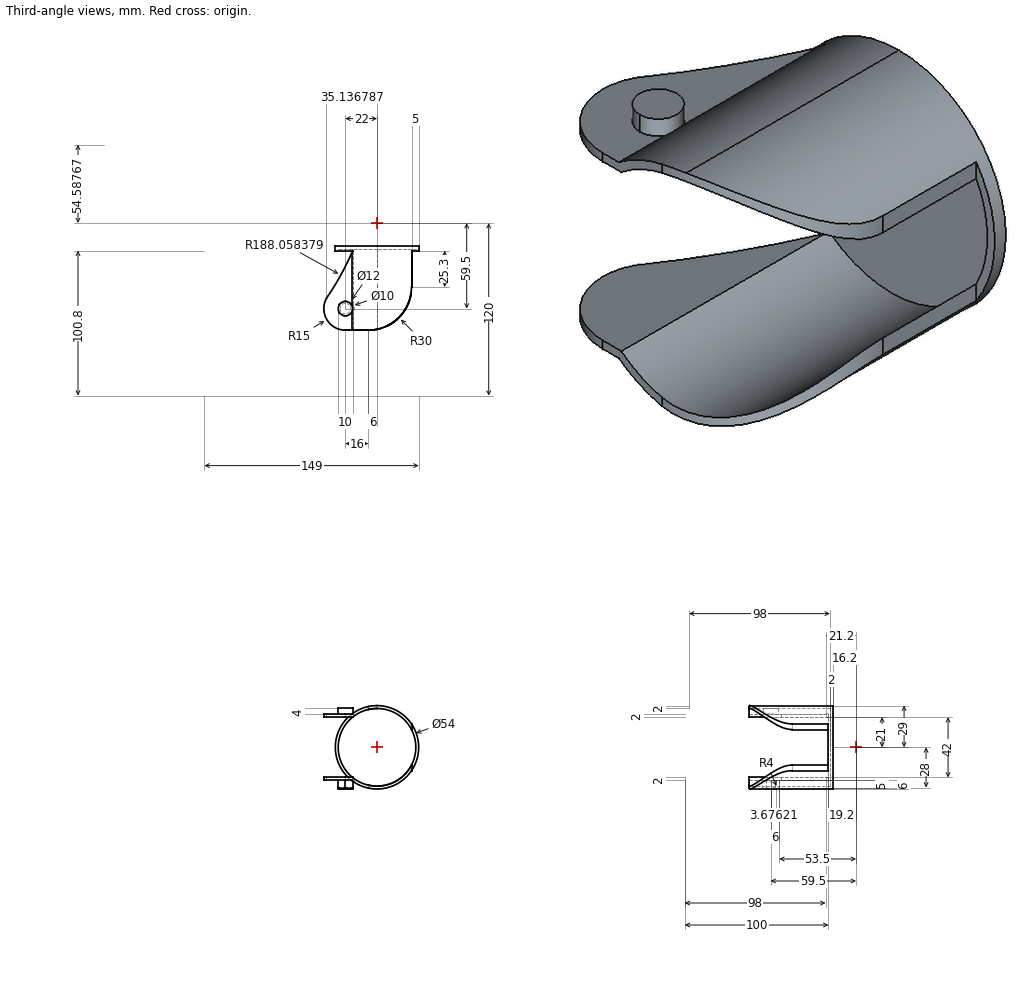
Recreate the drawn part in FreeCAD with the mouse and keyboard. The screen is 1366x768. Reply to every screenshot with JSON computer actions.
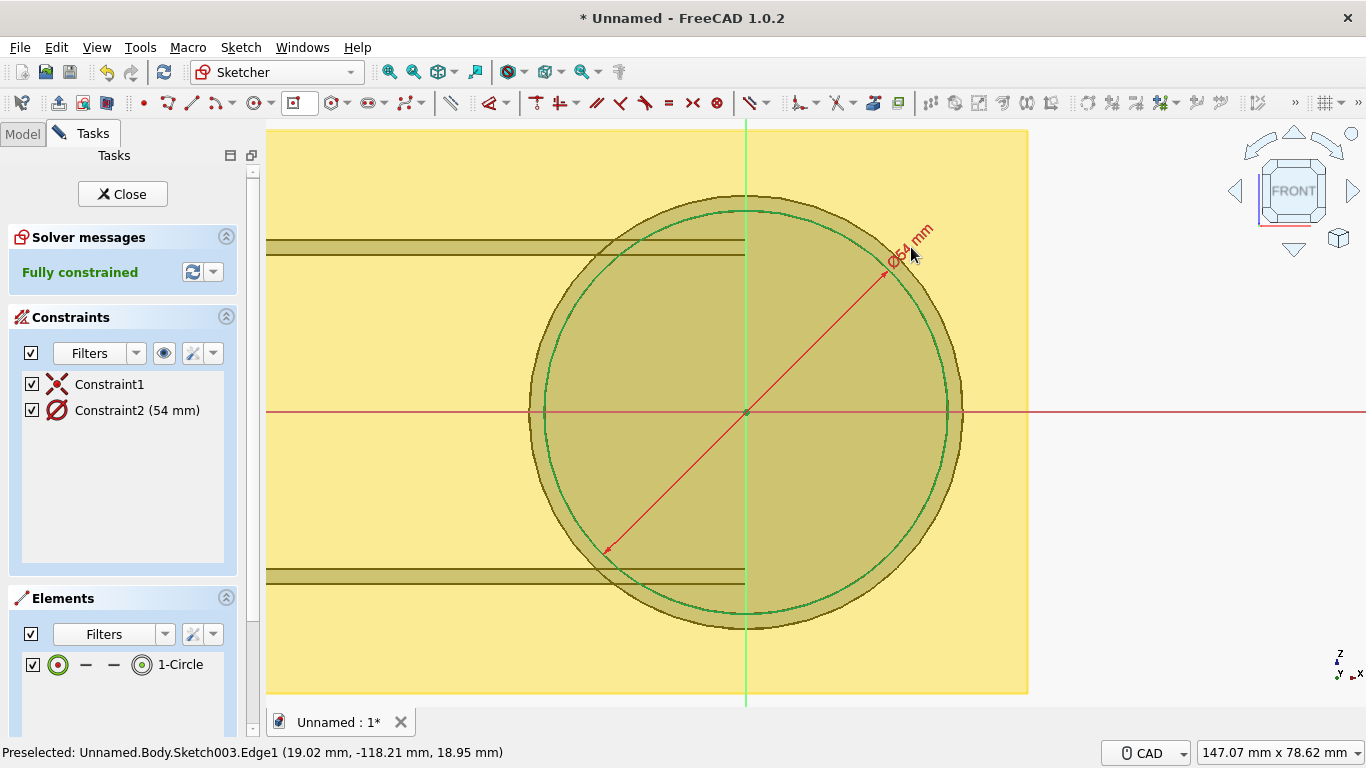
{"action": "left_click", "coordinate": [123, 194]}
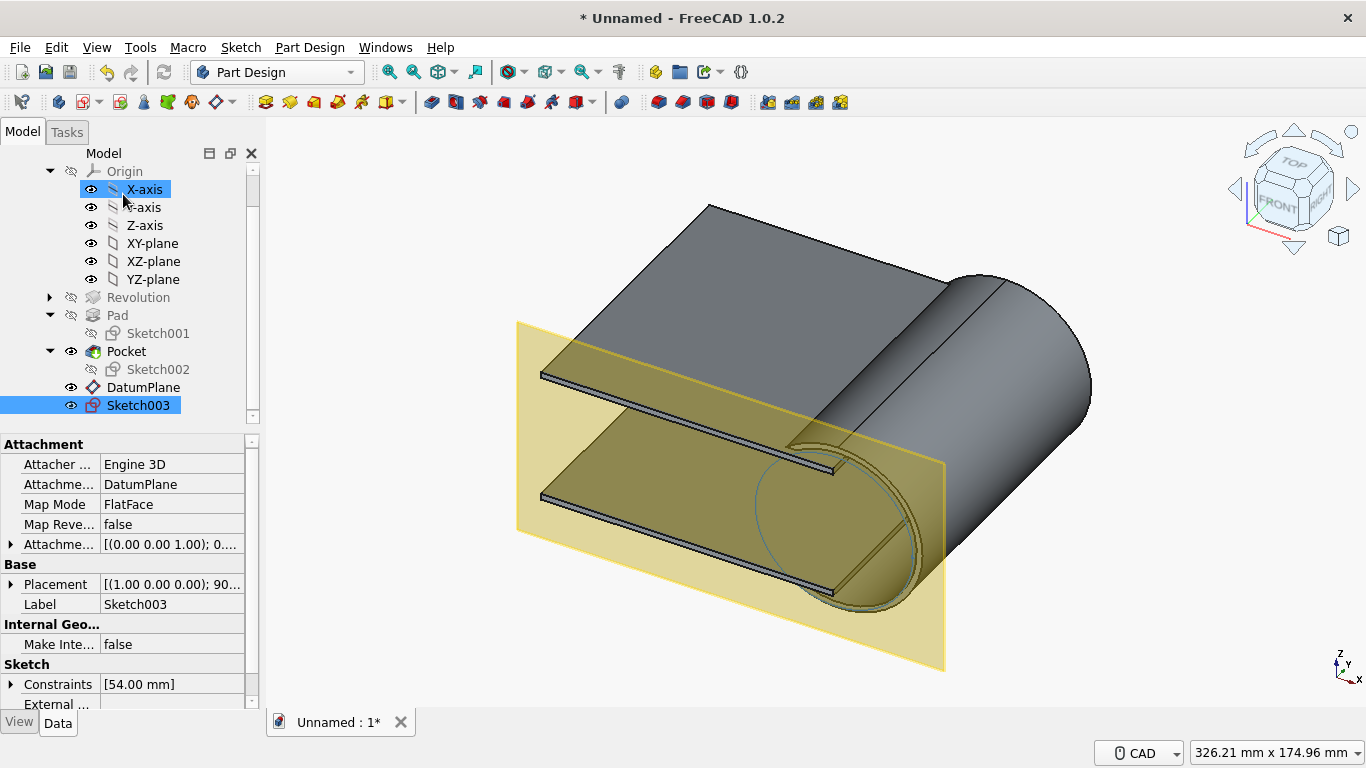
{"action": "left_click", "coordinate": [432, 102]}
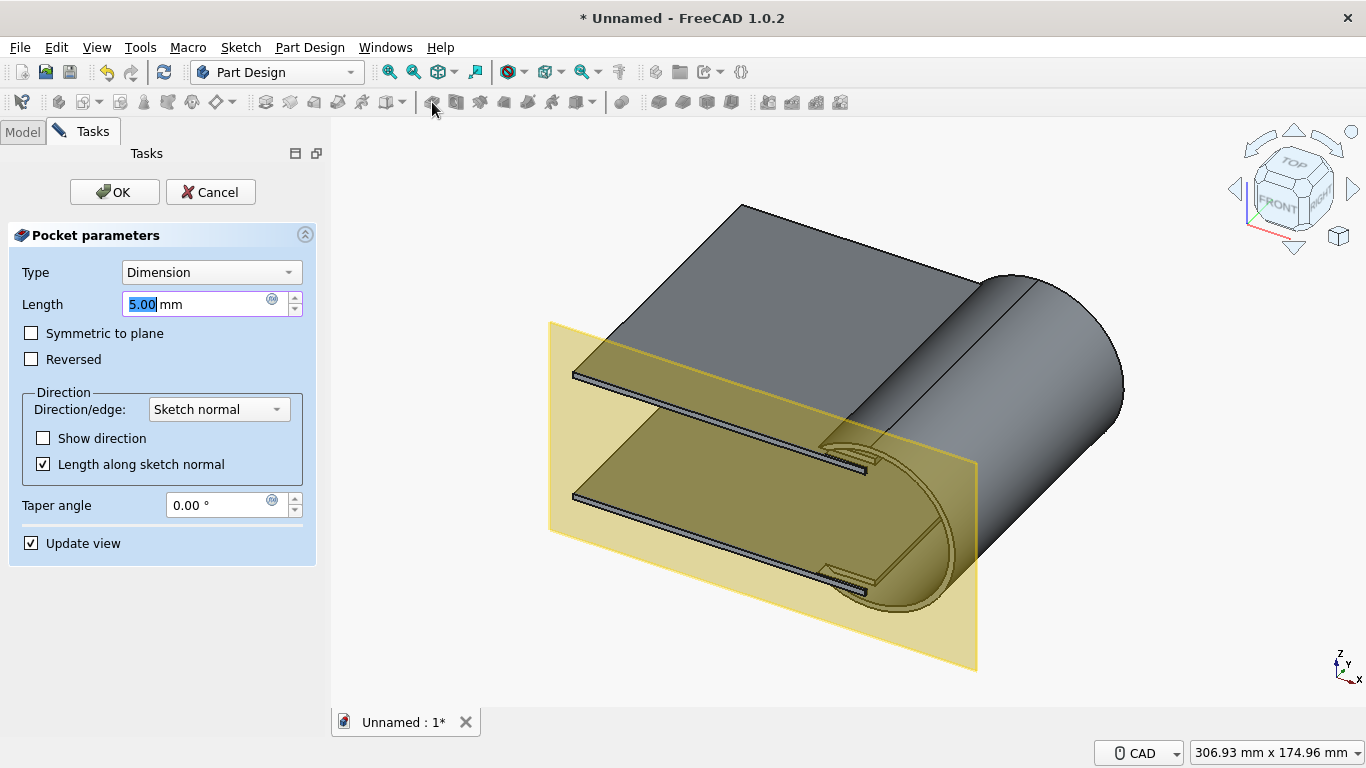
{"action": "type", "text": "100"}
{"action": "key", "text": "Tab"}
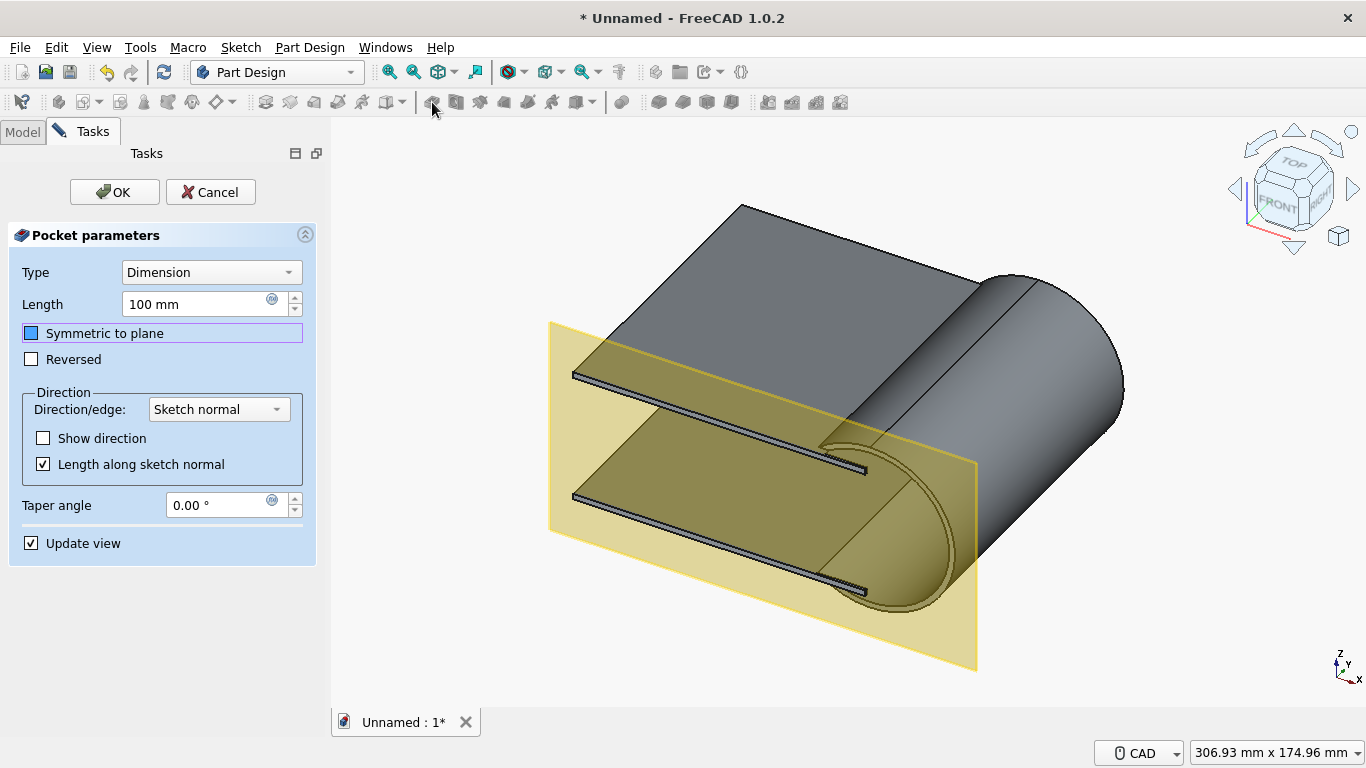
{"action": "left_click", "coordinate": [115, 192]}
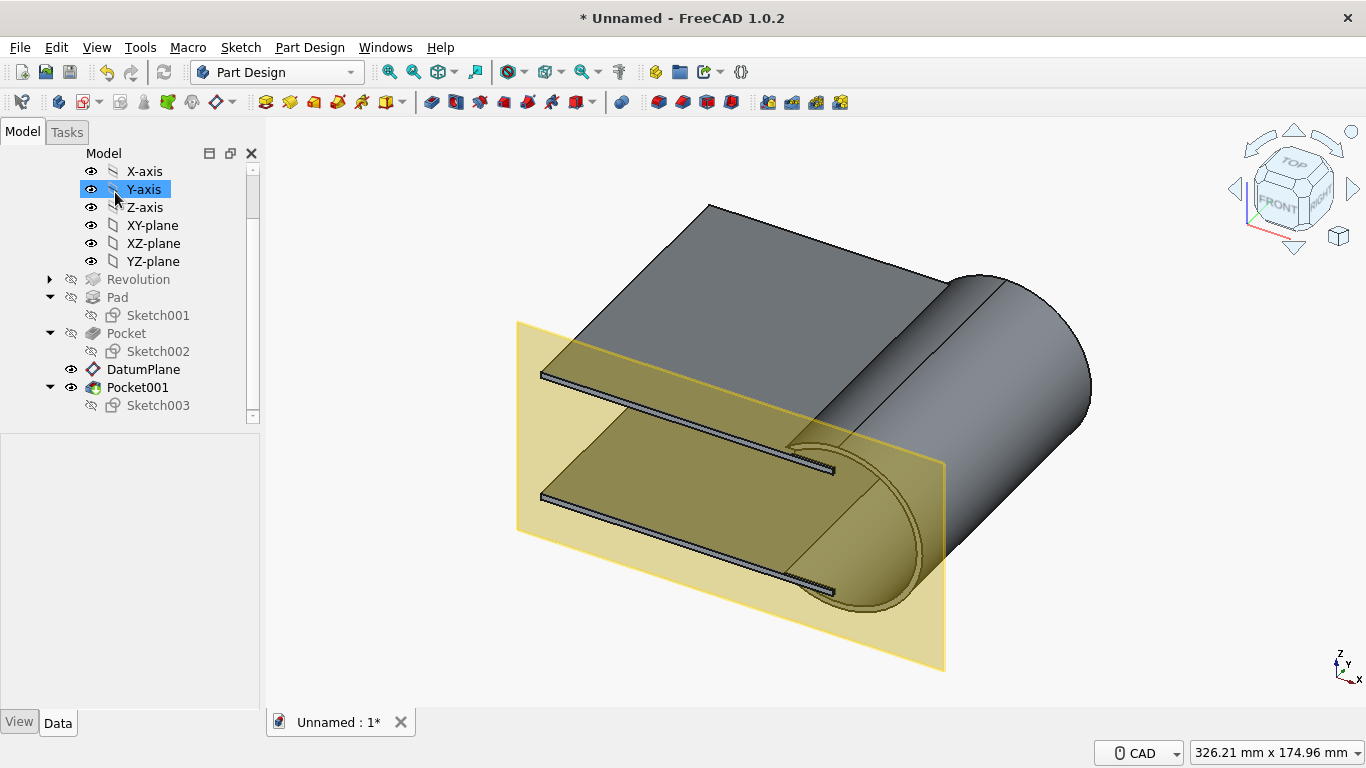
{"action": "left_click", "coordinate": [116, 369]}
{"action": "key", "text": "space"}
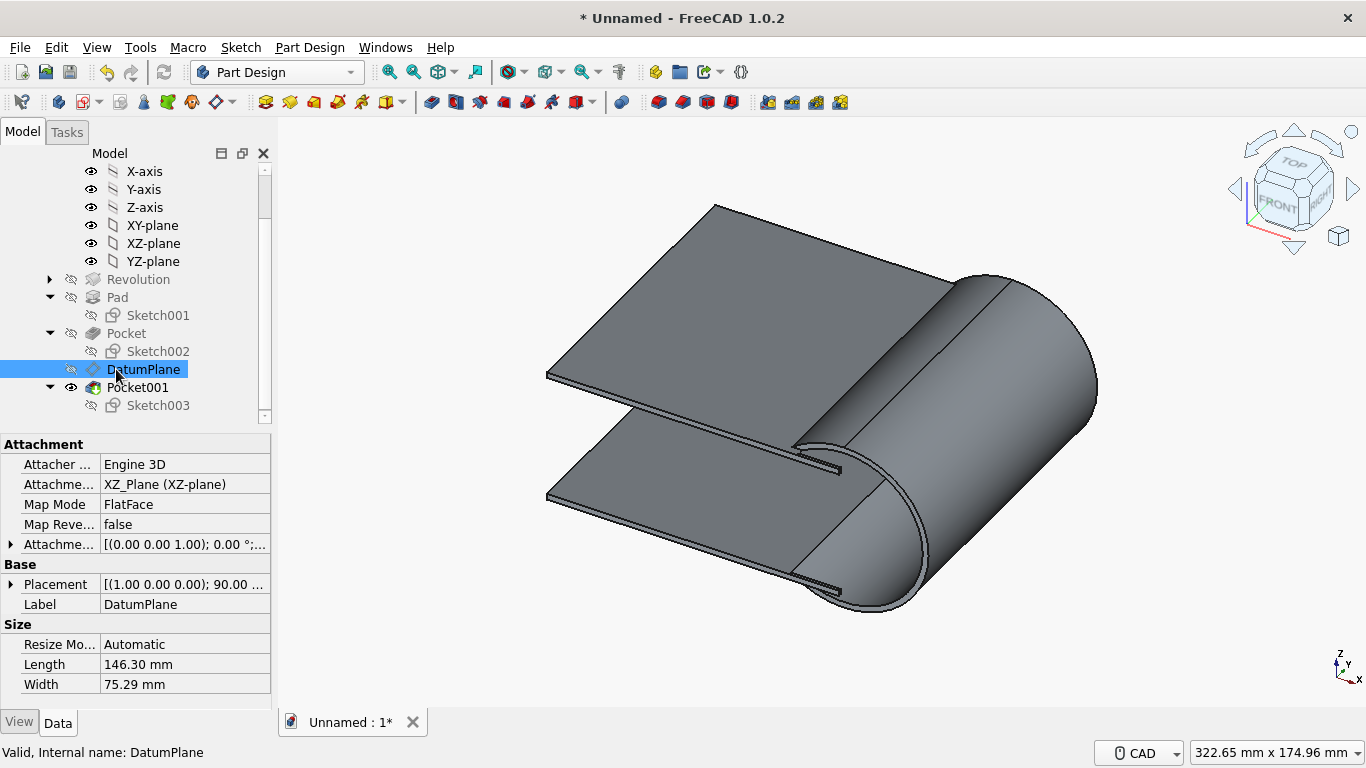
{"action": "left_click", "coordinate": [318, 667]}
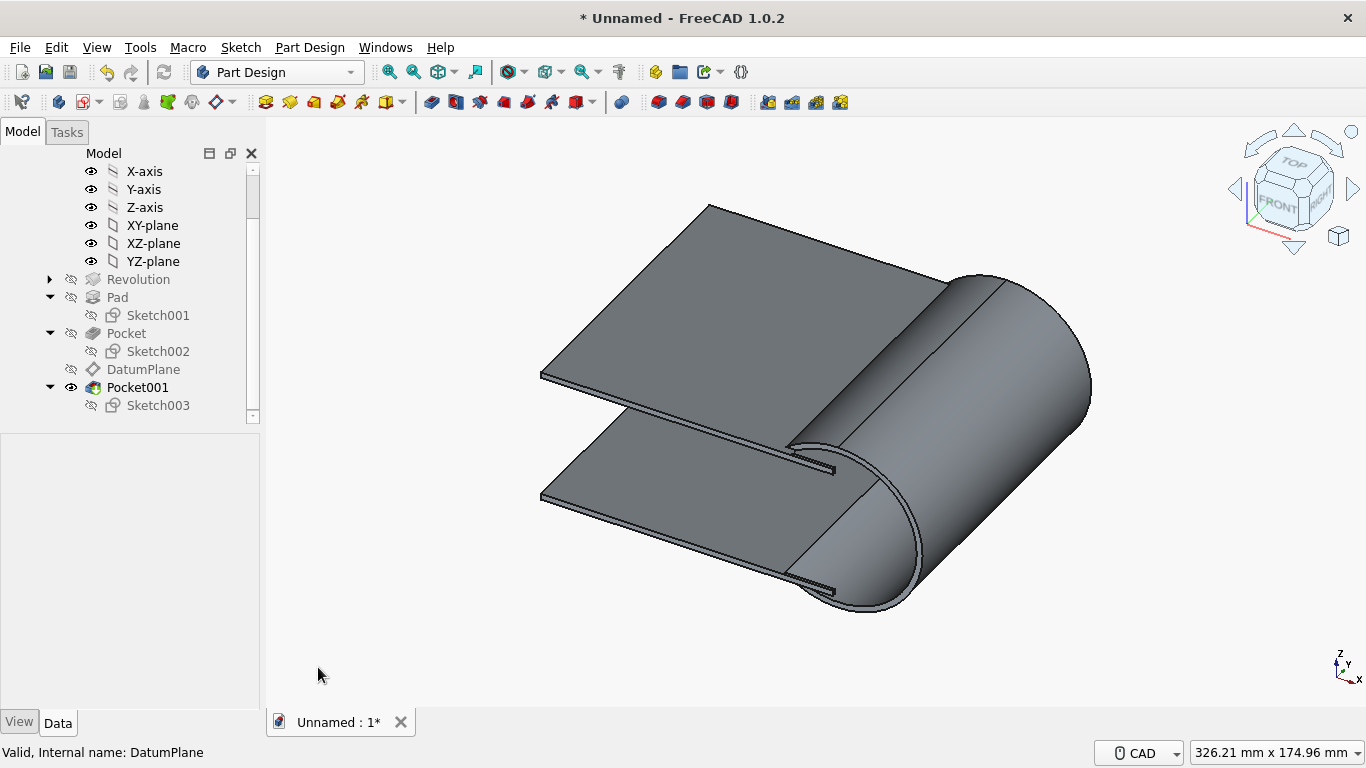
{"action": "left_click", "coordinate": [84, 102]}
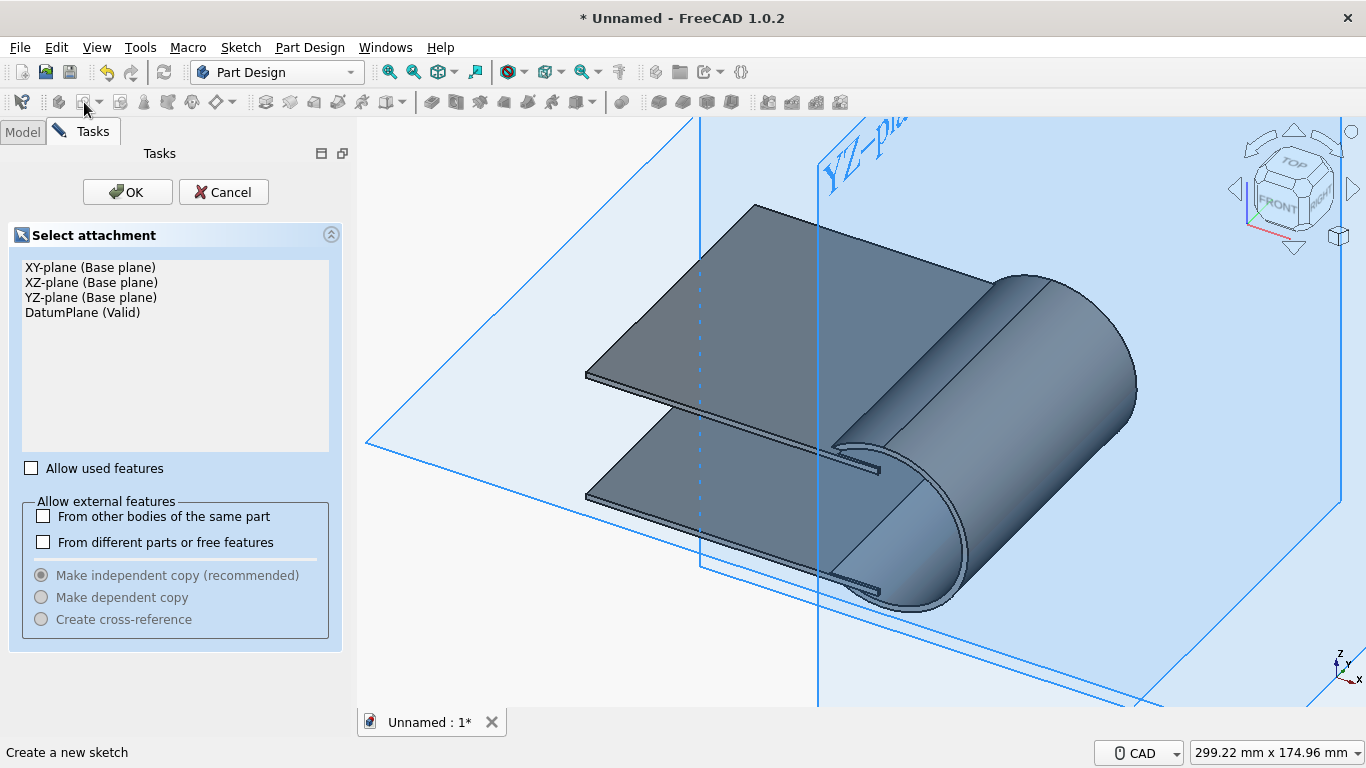
{"action": "left_click", "coordinate": [82, 268]}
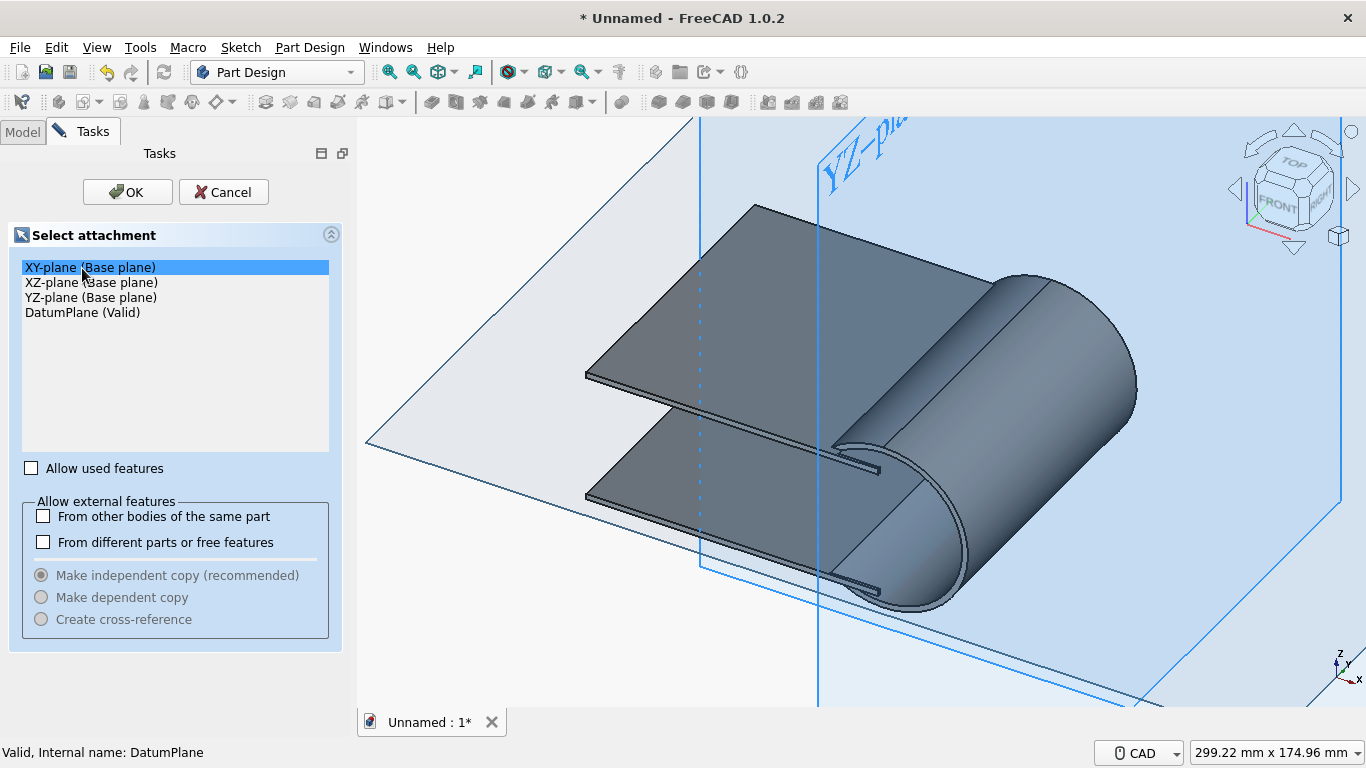
{"action": "left_click", "coordinate": [128, 192]}